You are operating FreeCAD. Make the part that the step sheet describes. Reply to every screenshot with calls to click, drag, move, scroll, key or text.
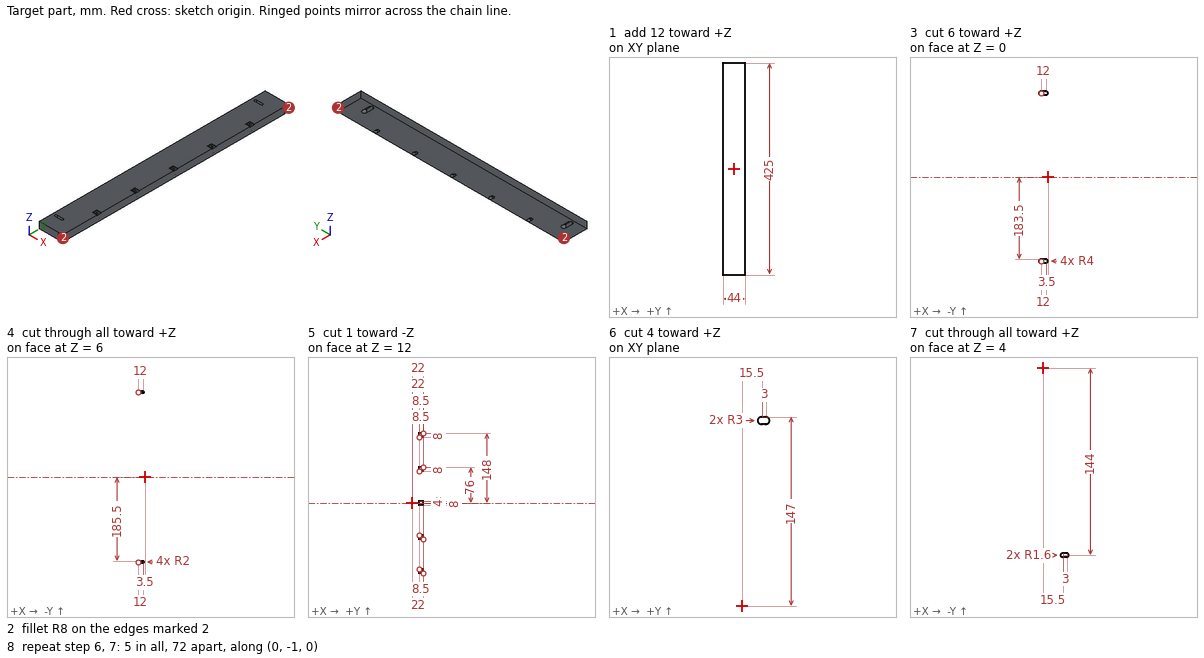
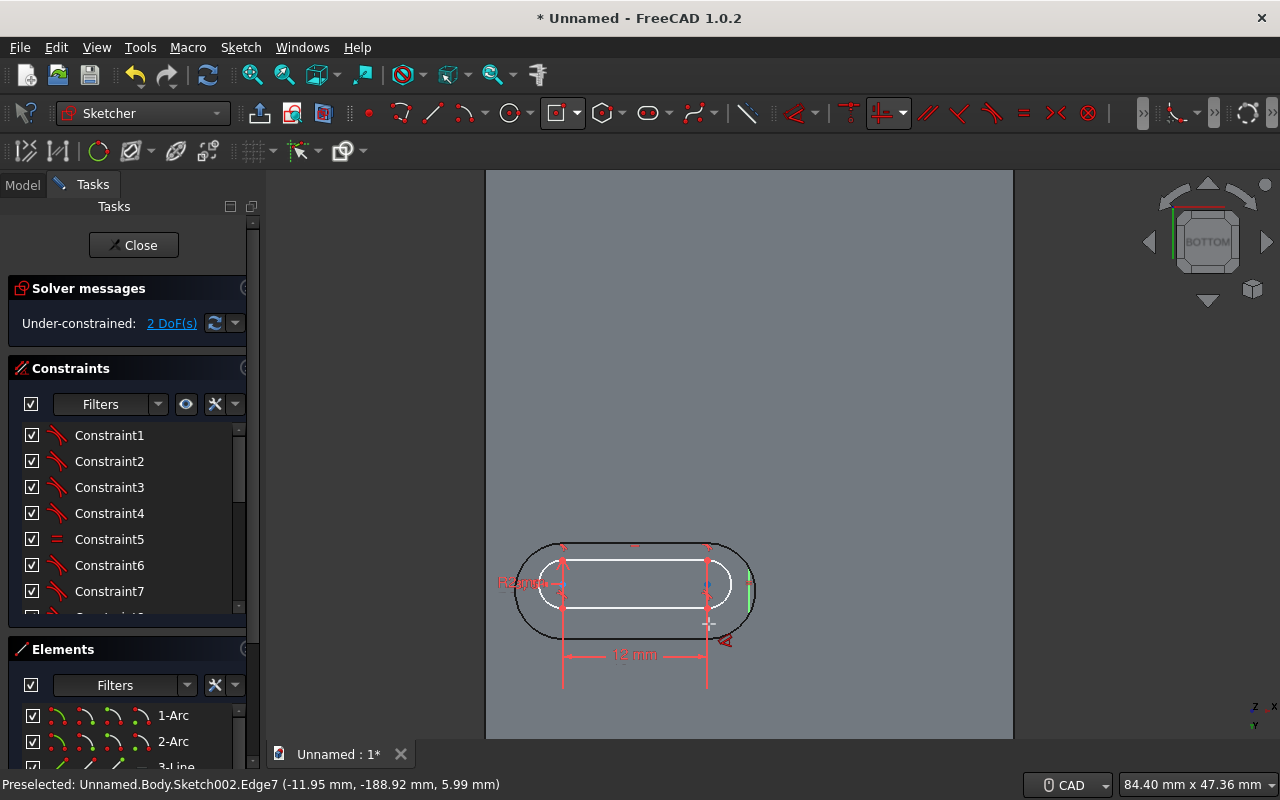
click(707, 608)
click(728, 642)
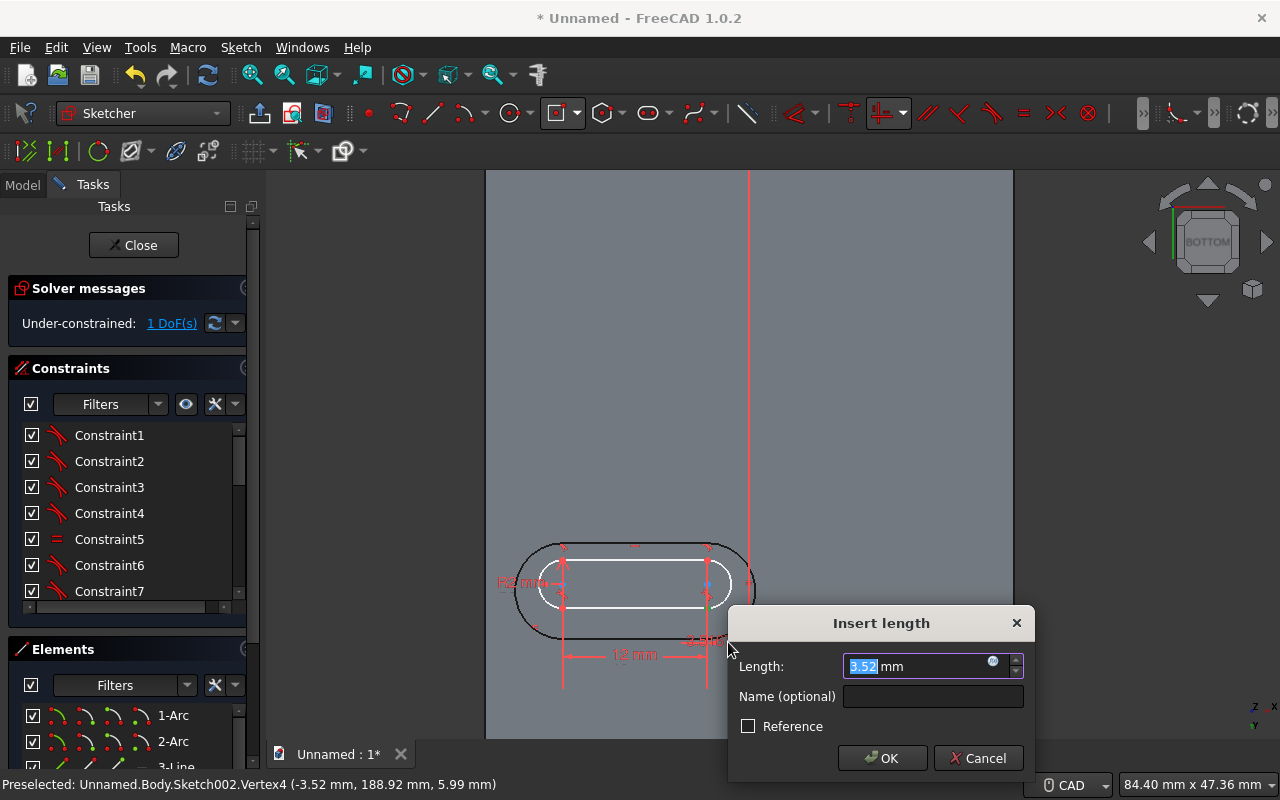
text(3.5)
key(Return)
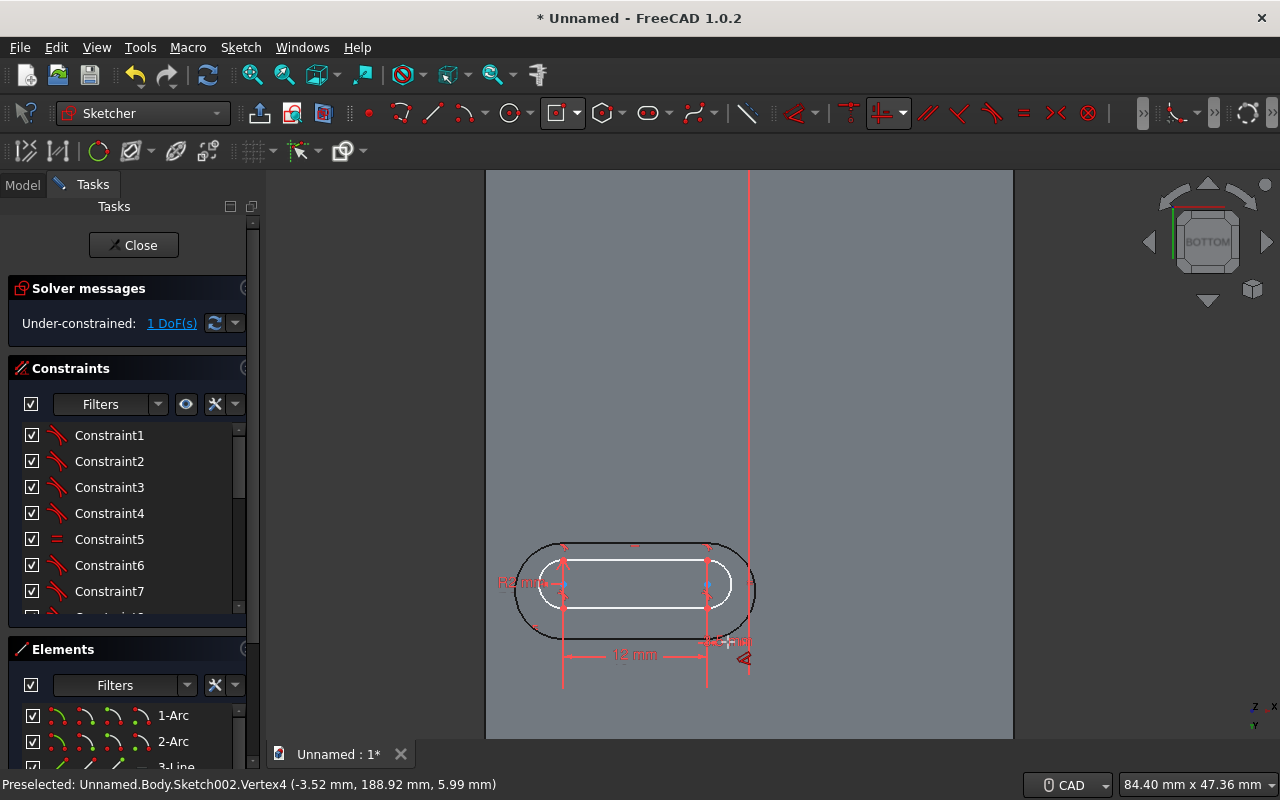
click(563, 560)
click(783, 379)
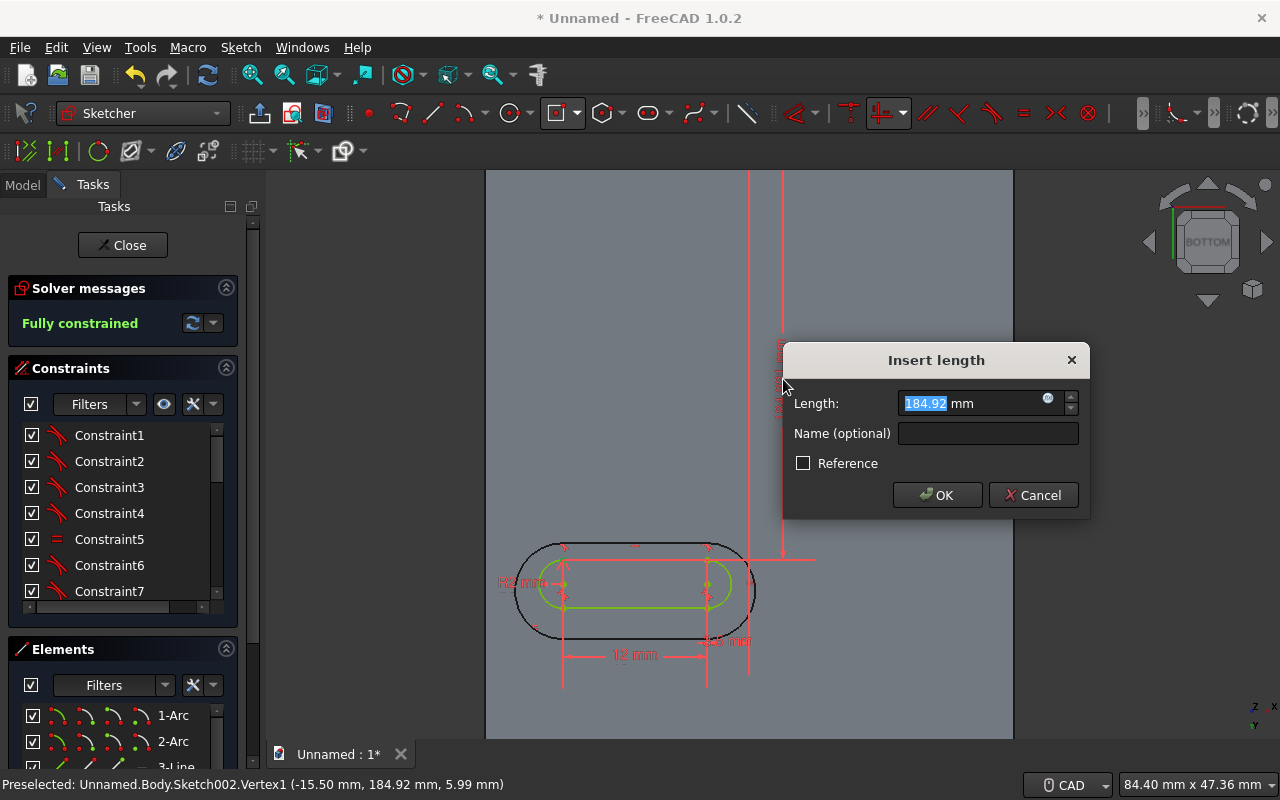
text(185.5)
key(Return)
key(Escape)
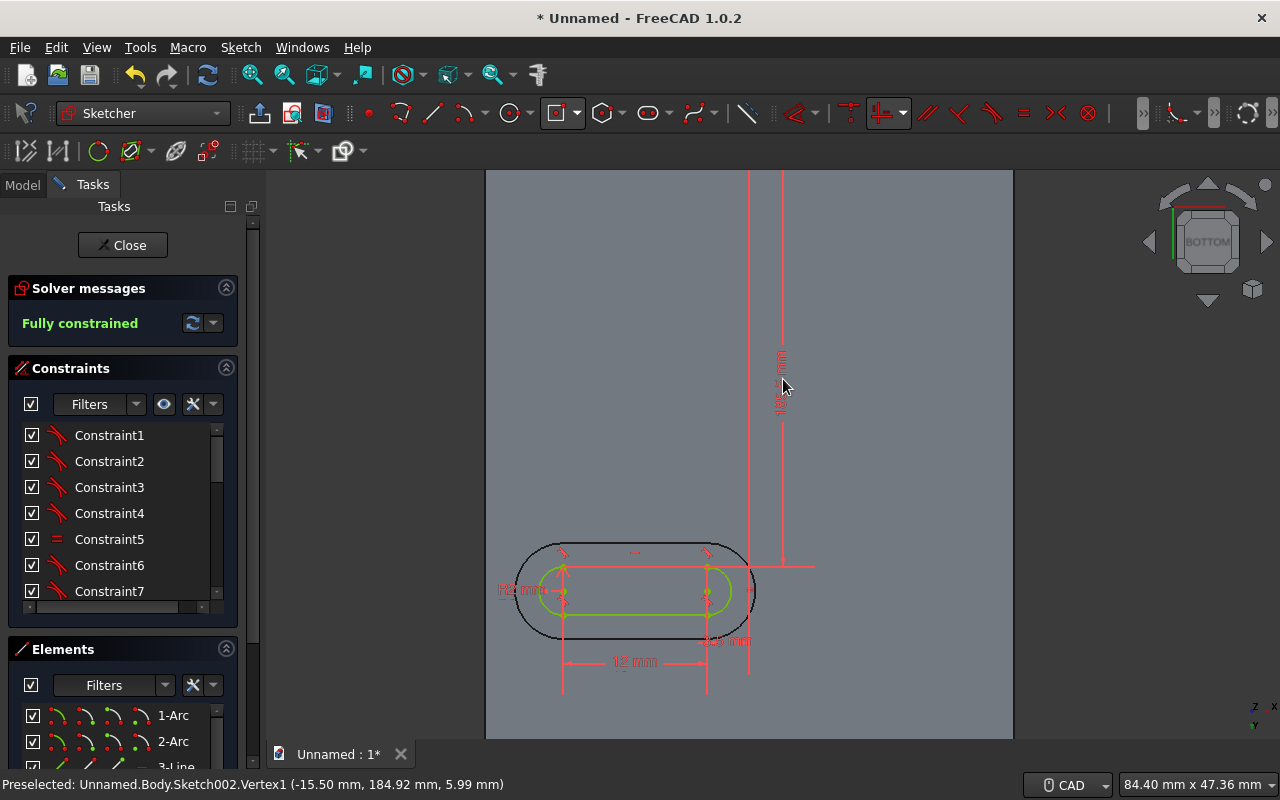
click(123, 245)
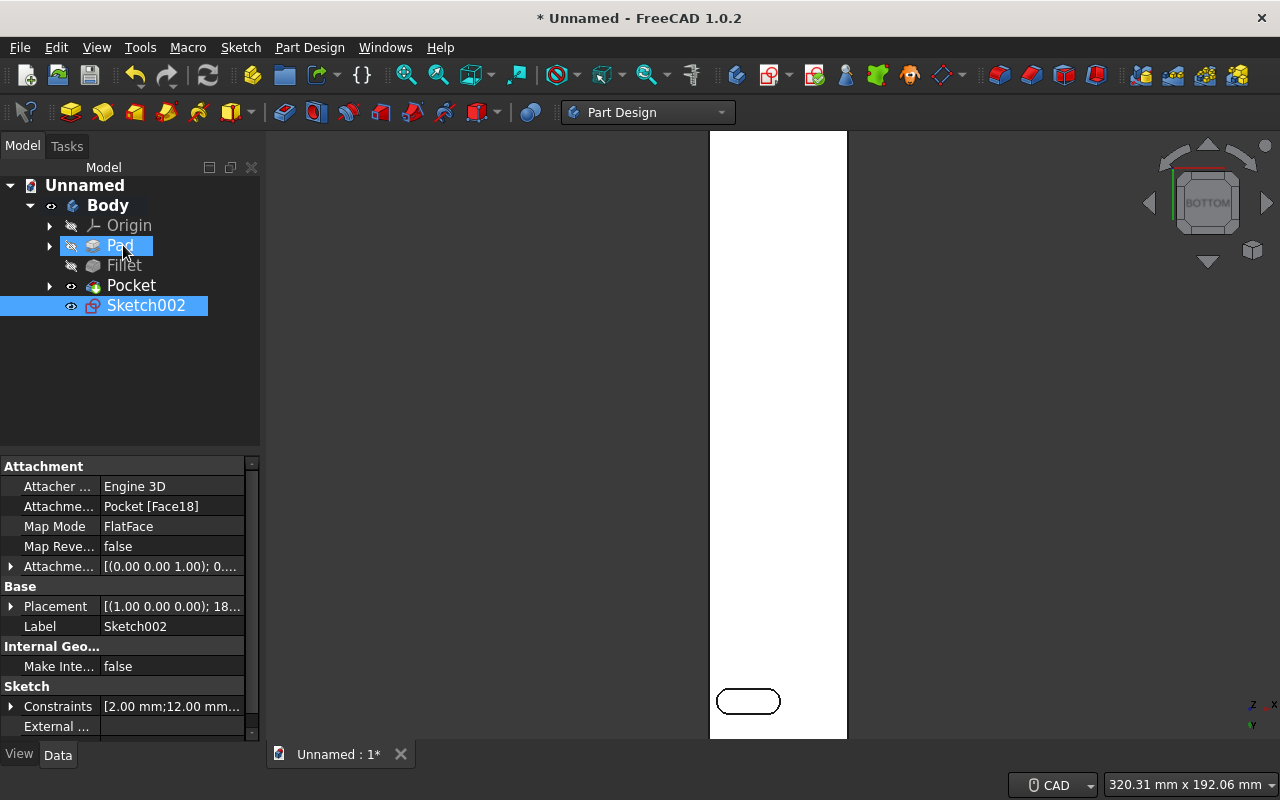
click(286, 112)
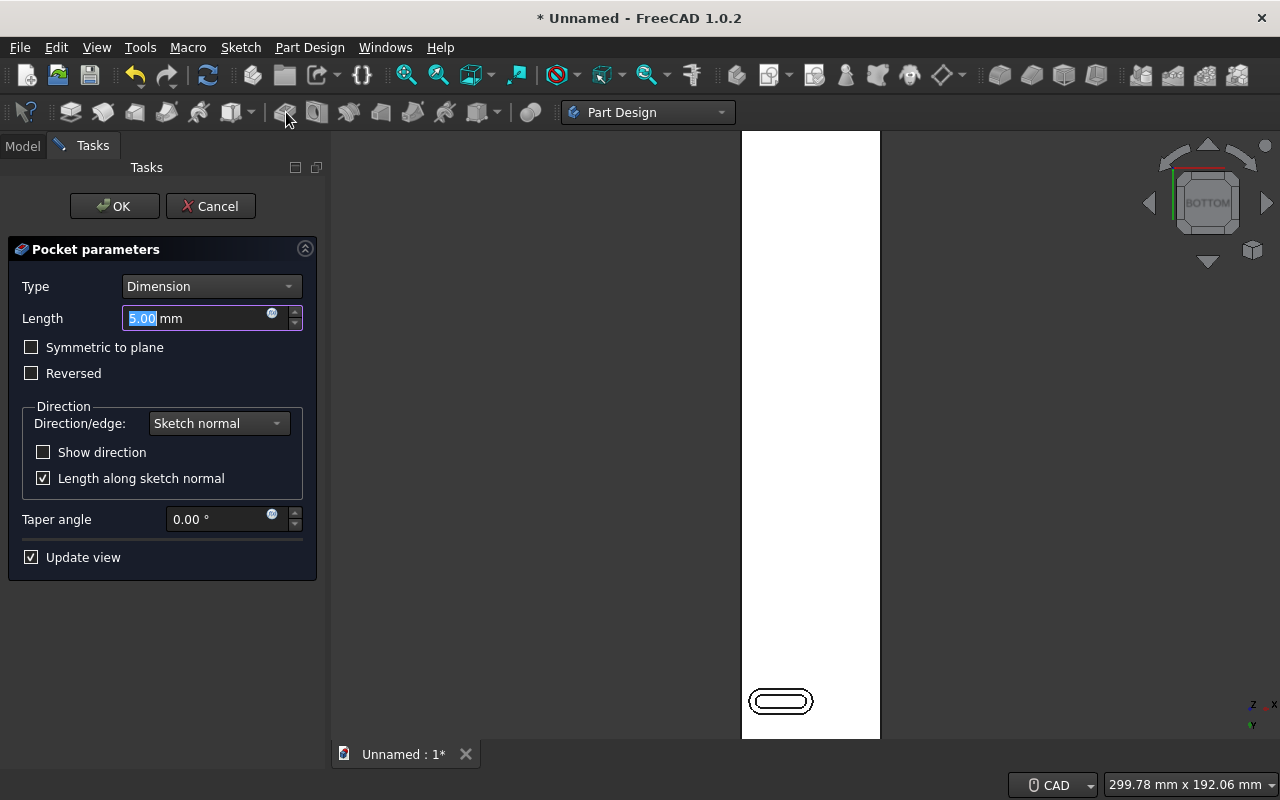
click(212, 286)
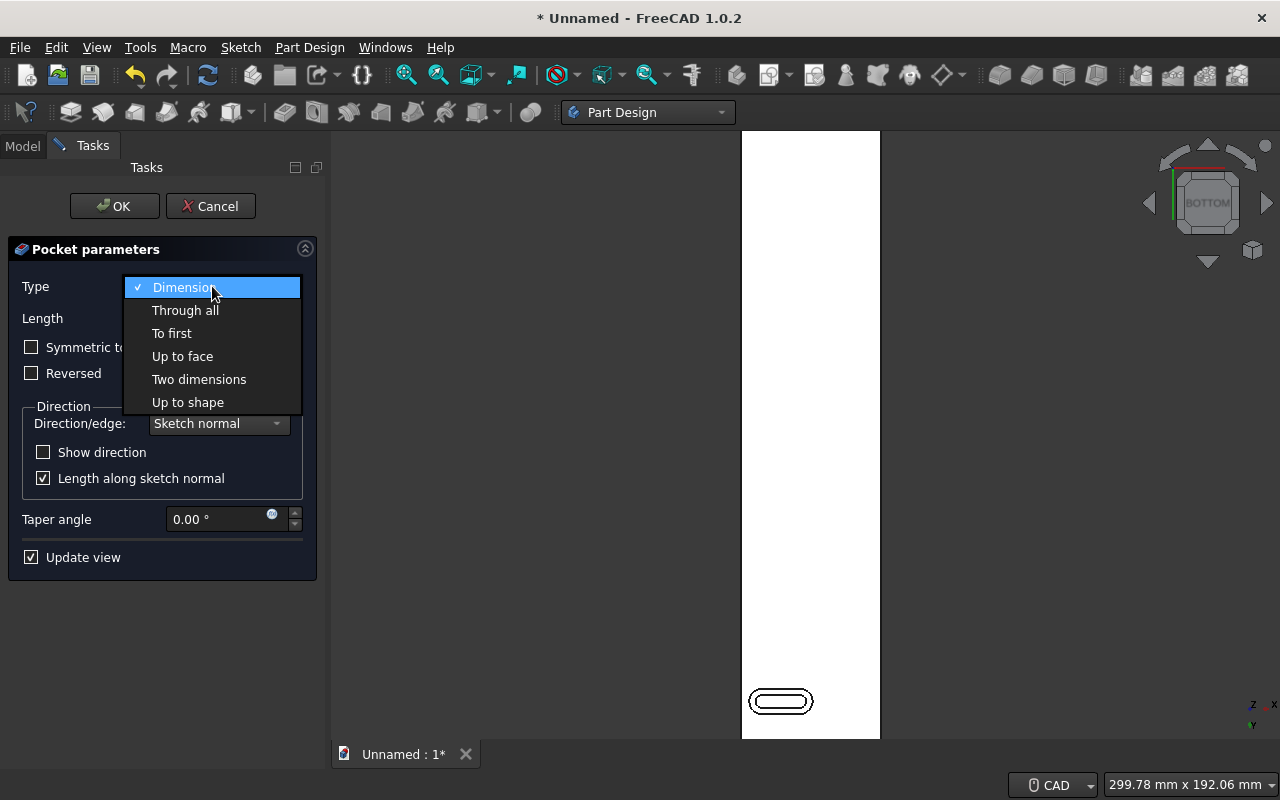
click(212, 310)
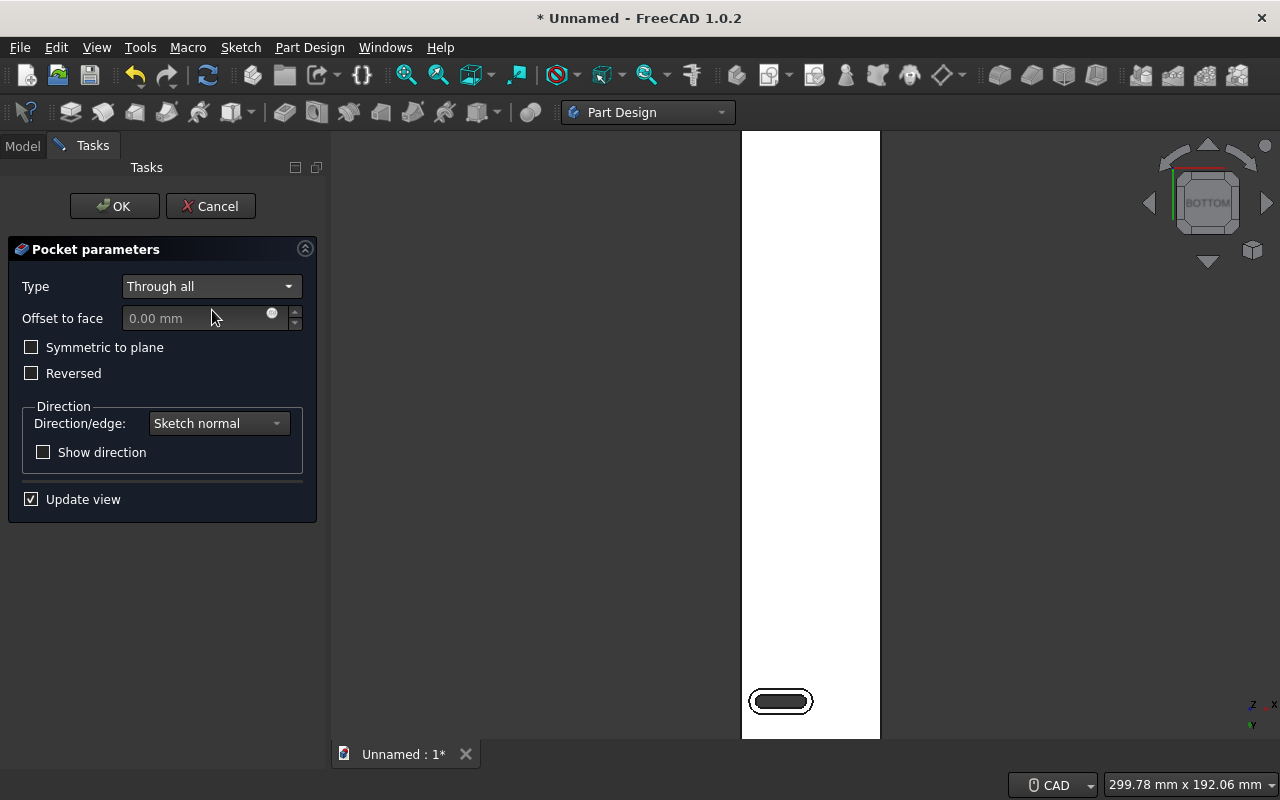
click(115, 206)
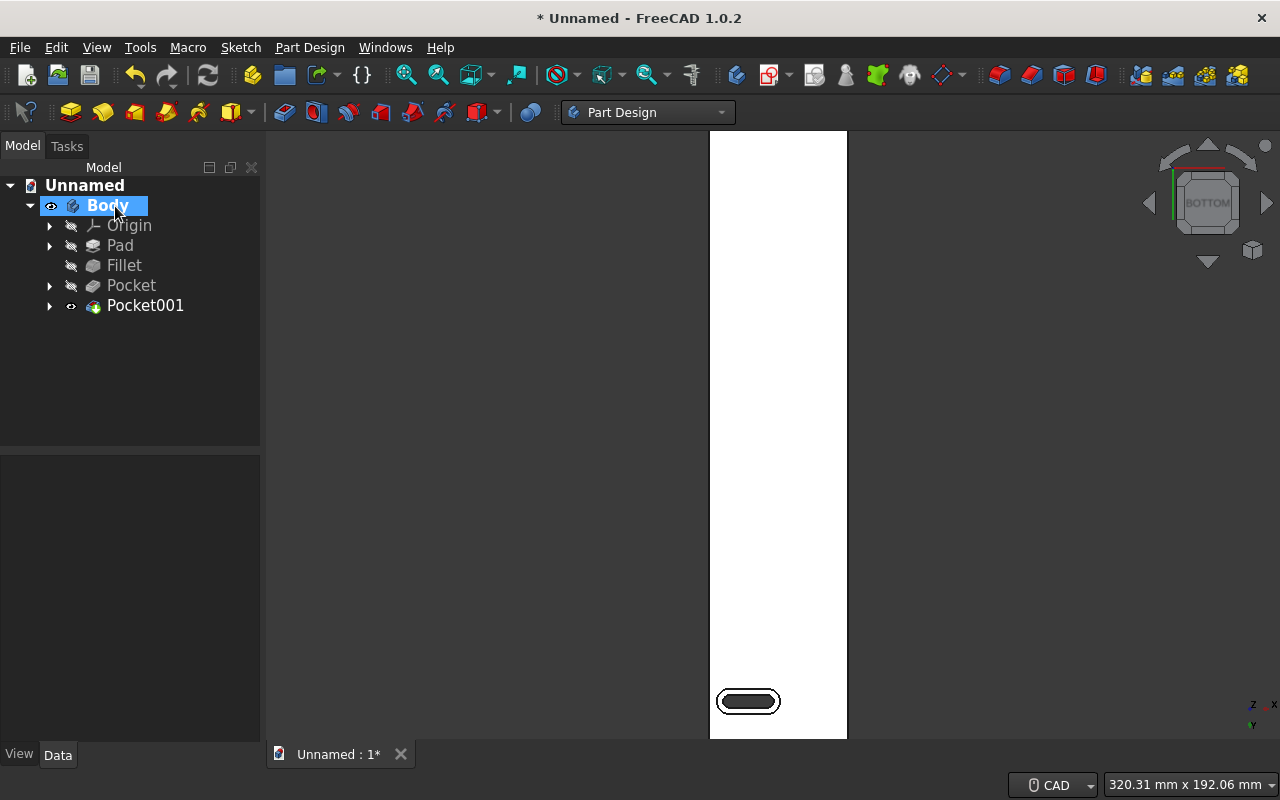
click(408, 76)